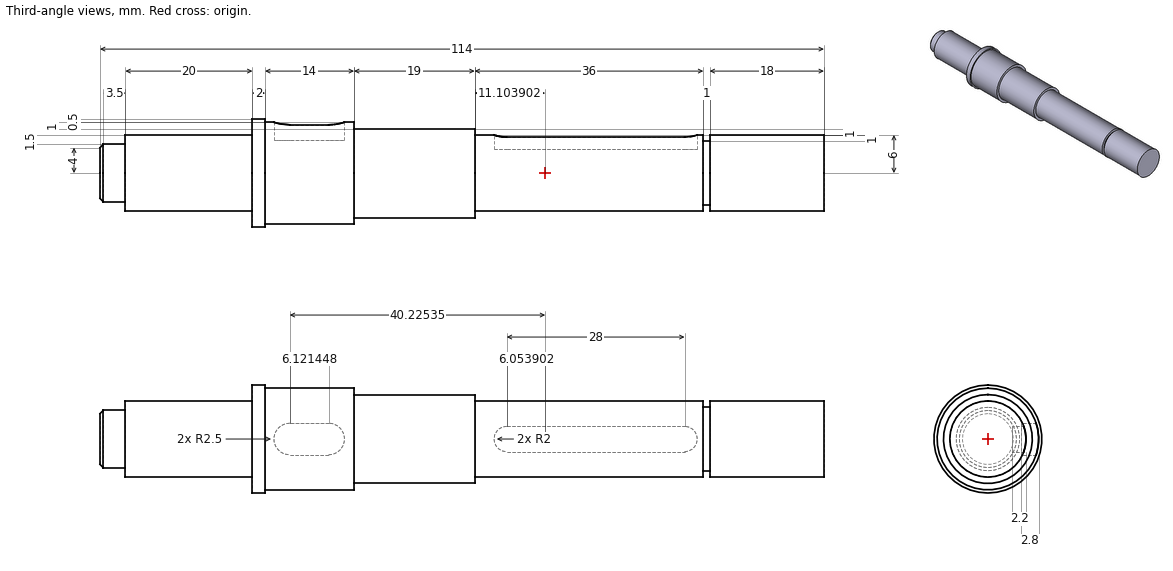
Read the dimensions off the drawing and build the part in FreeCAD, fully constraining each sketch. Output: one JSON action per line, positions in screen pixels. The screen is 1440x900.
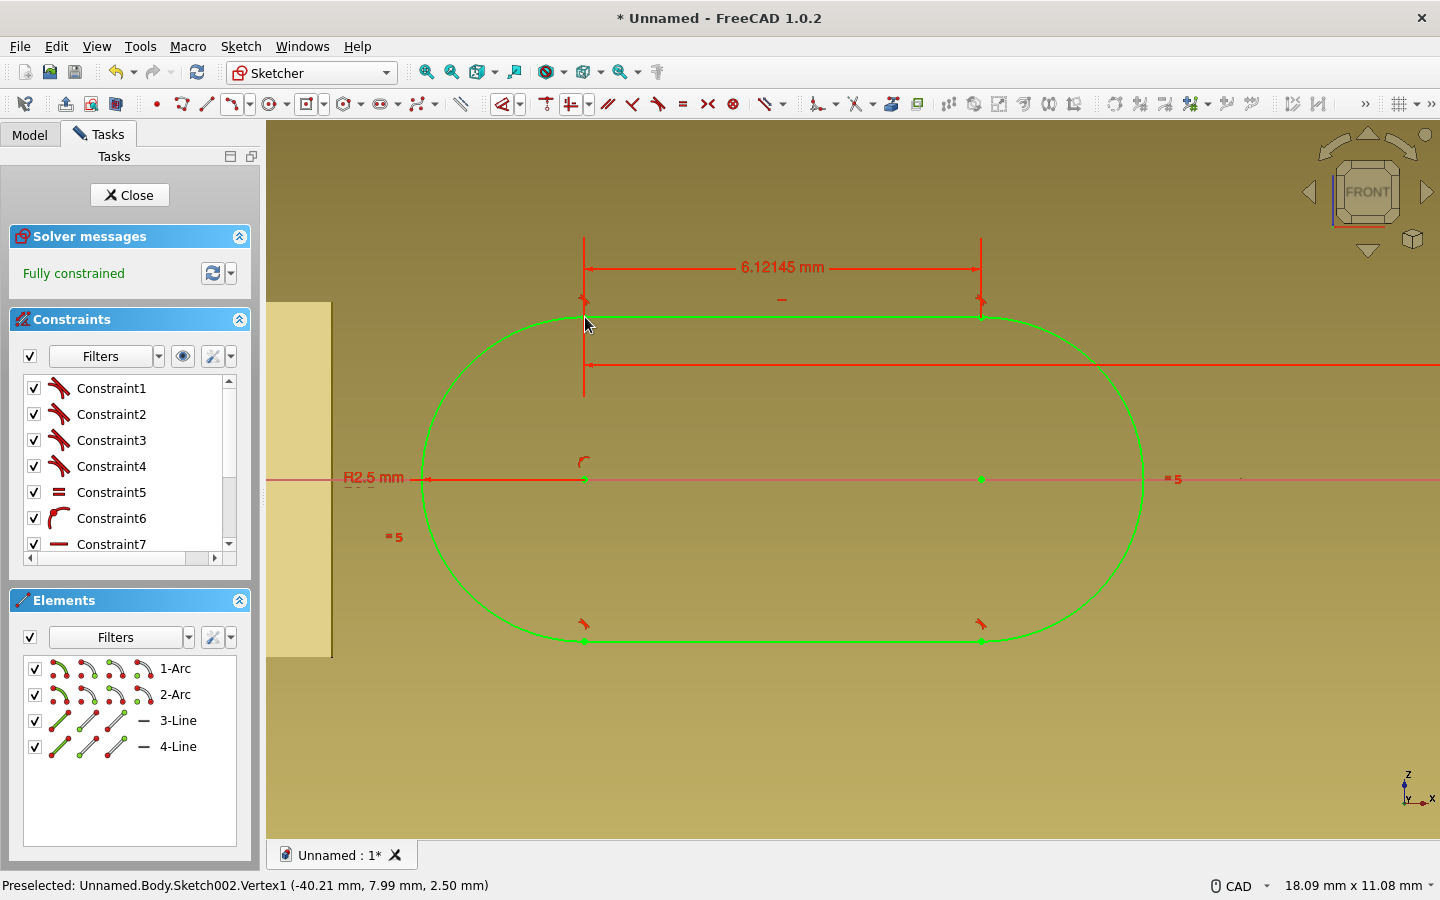
{"action": "left_click", "coordinate": [130, 195]}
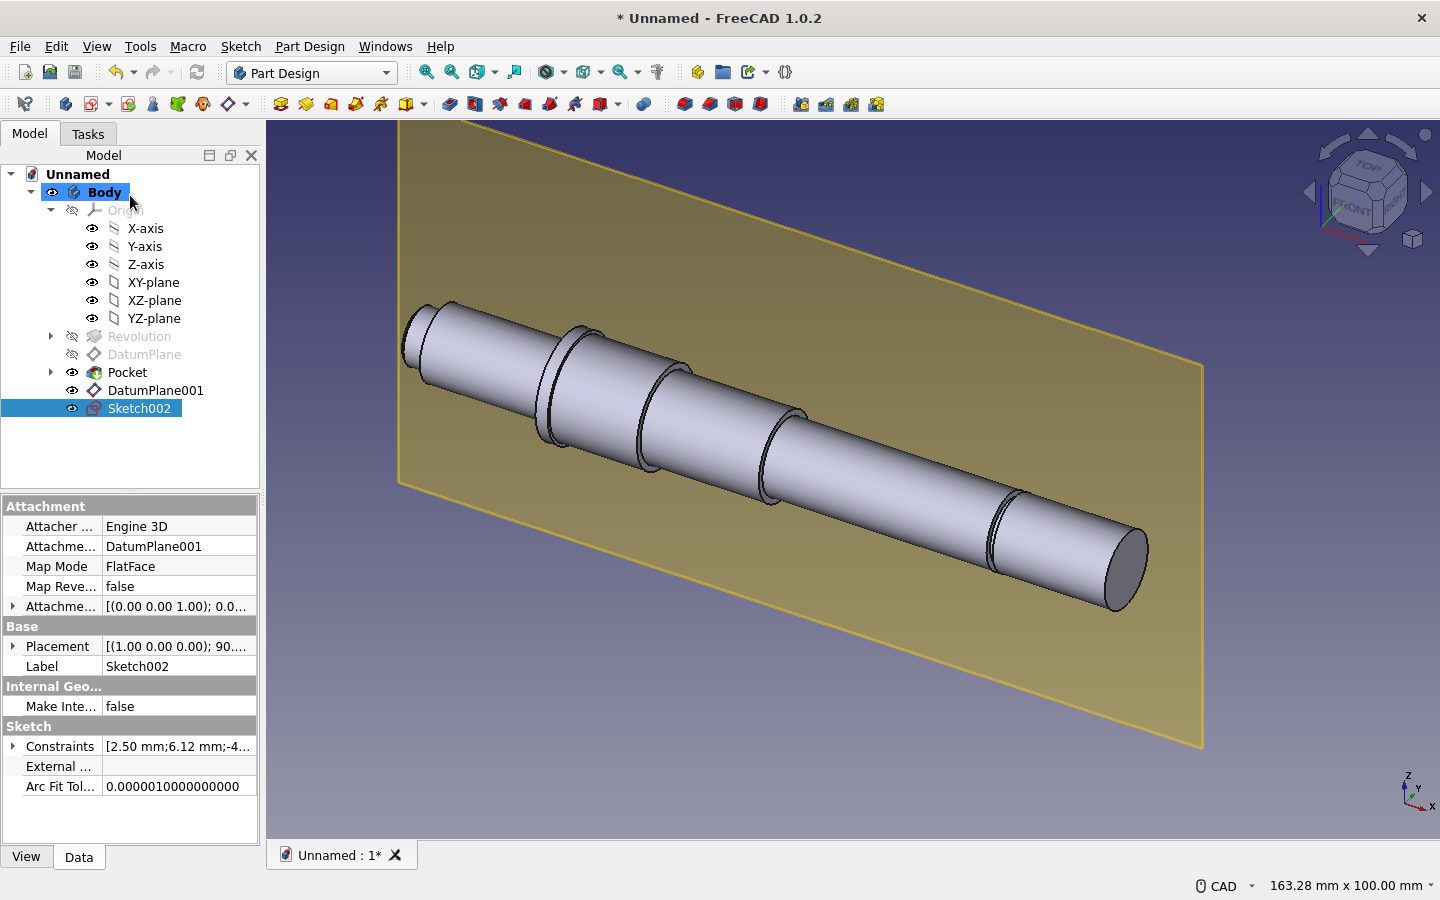
{"action": "left_click", "coordinate": [450, 104]}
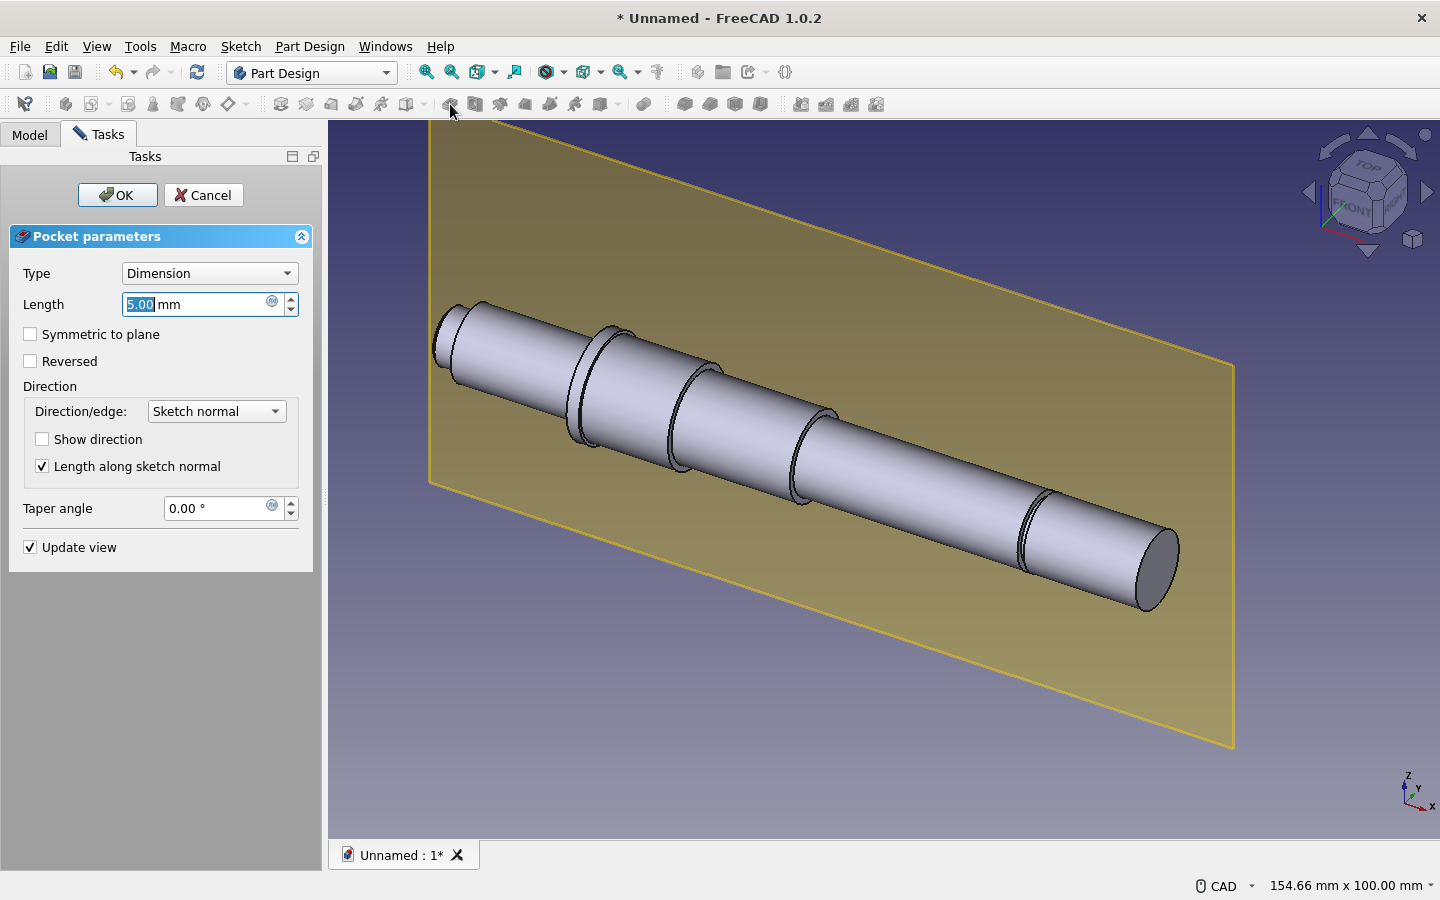
{"action": "type", "text": "2.8"}
{"action": "key", "text": "Tab"}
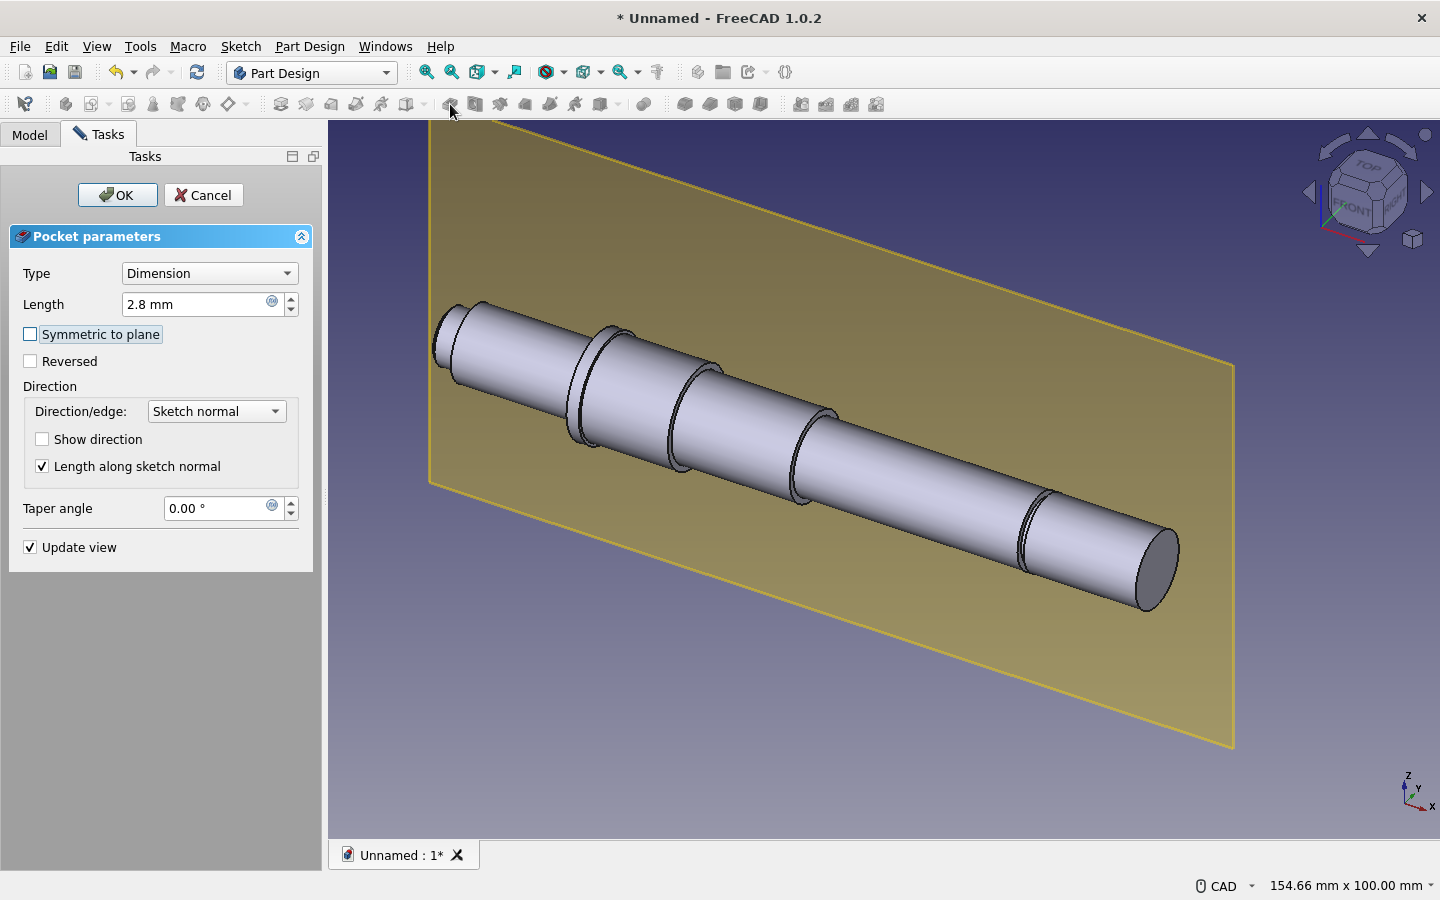
{"action": "left_click", "coordinate": [31, 361]}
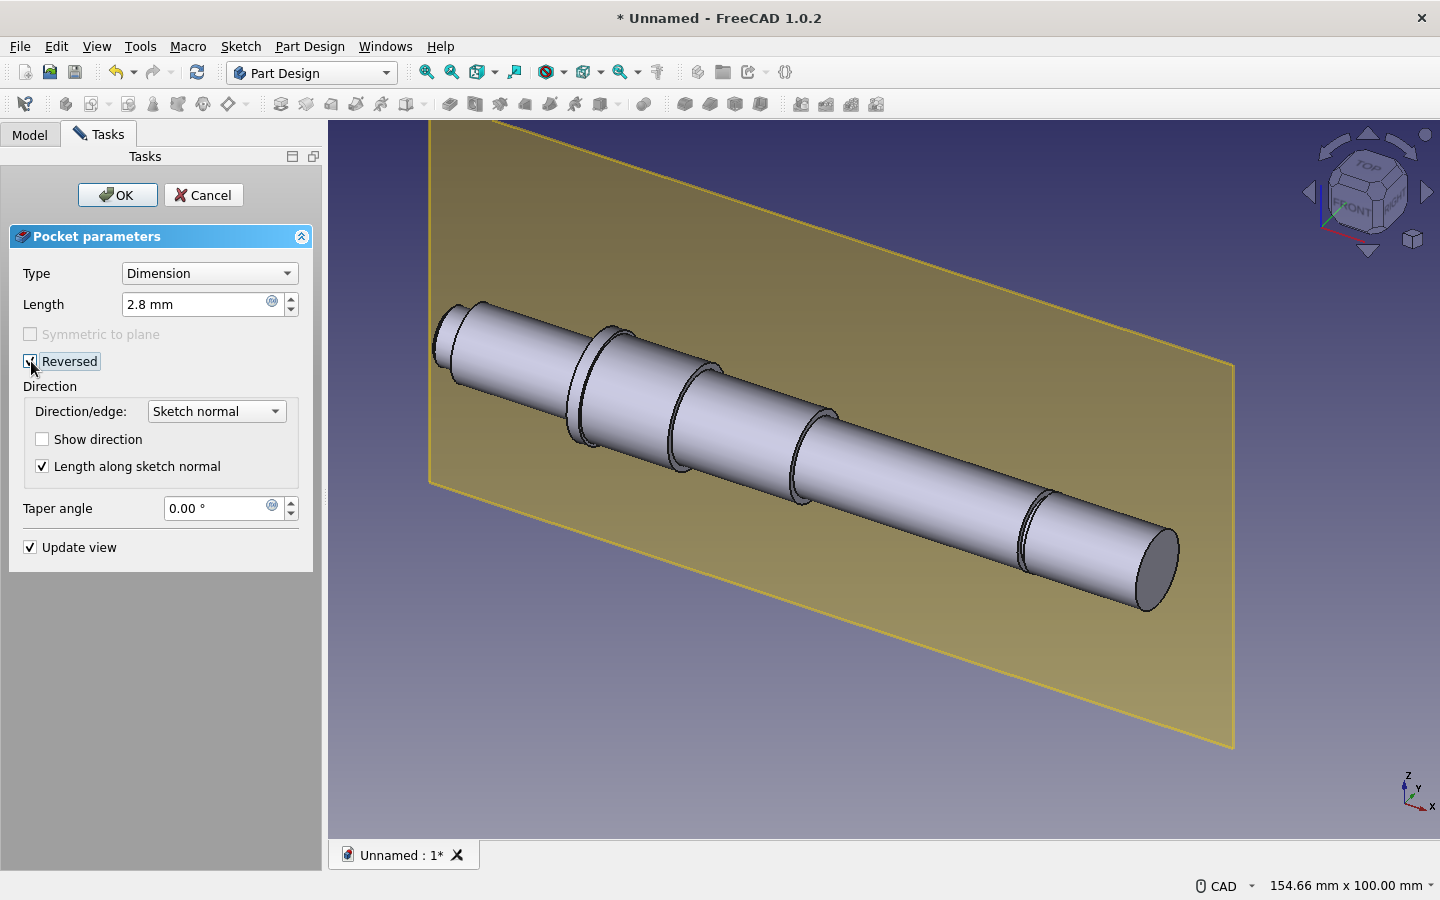
{"action": "left_click", "coordinate": [118, 195]}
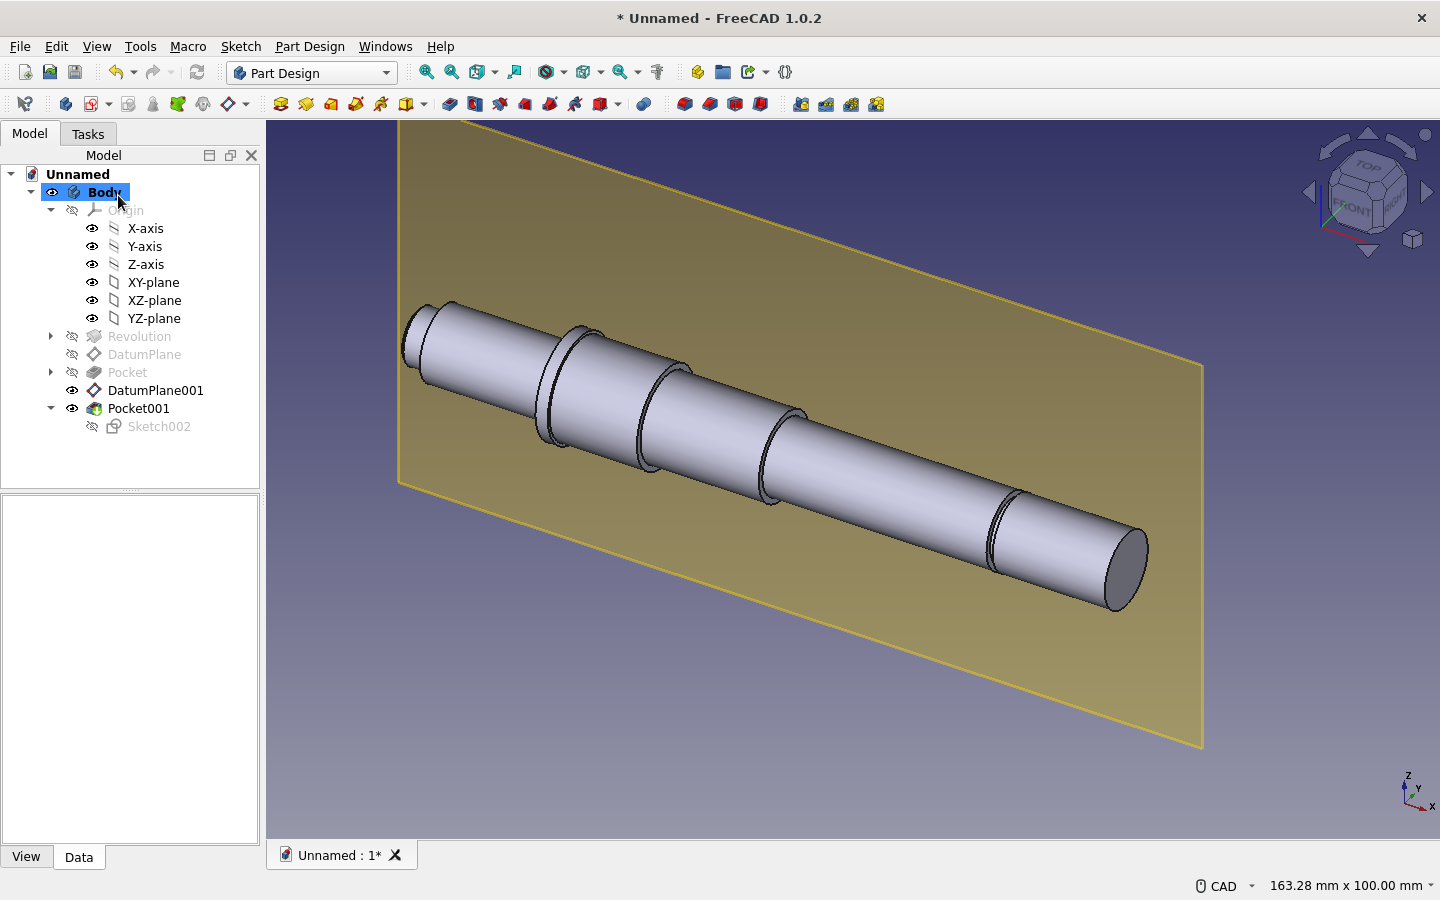
{"action": "left_click", "coordinate": [117, 390]}
{"action": "key", "text": "space"}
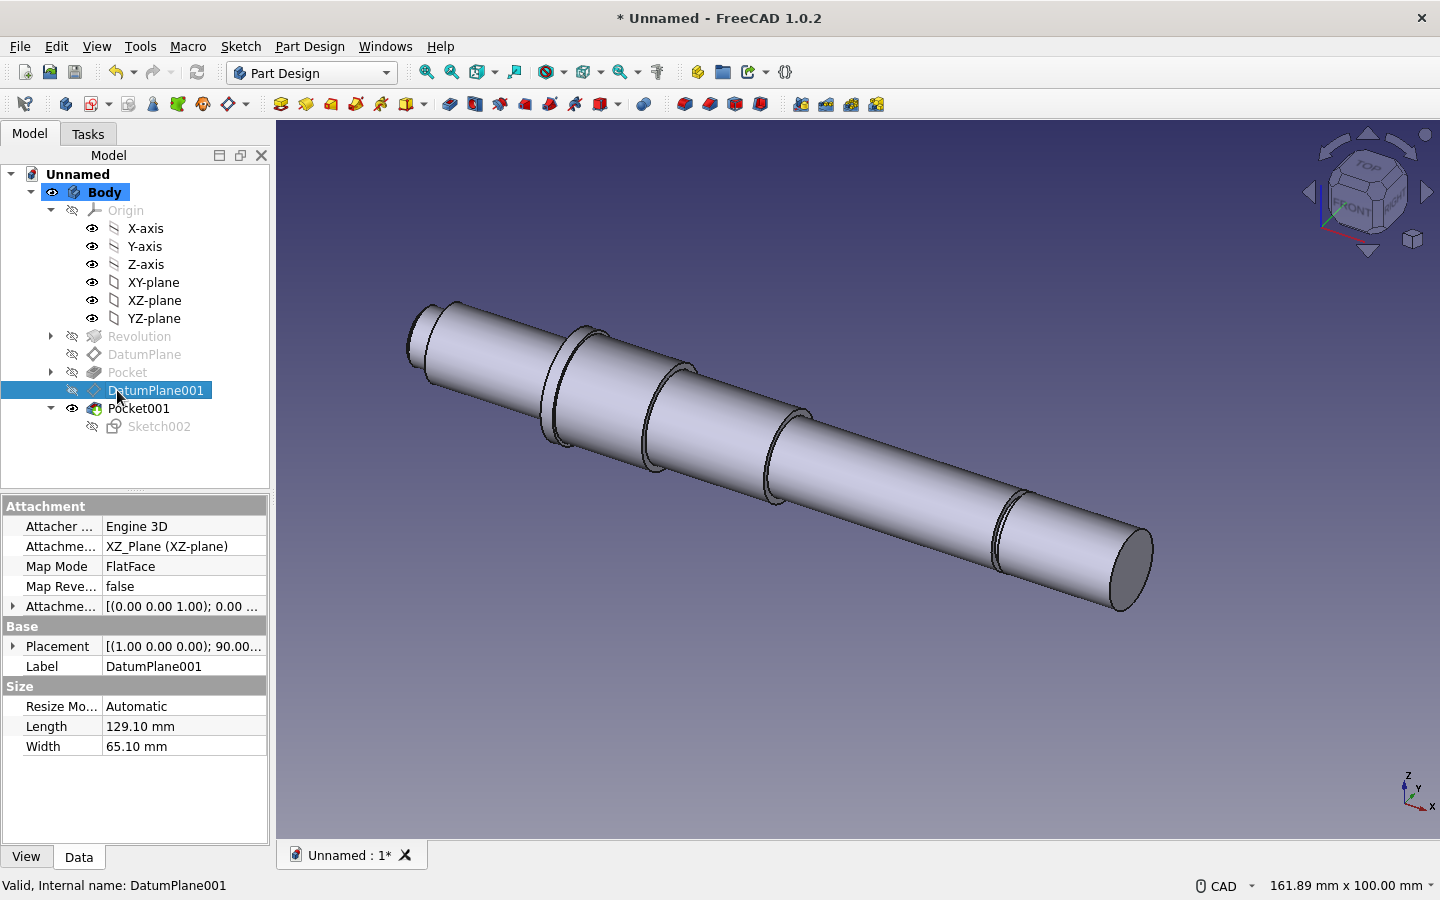
{"action": "key", "text": "0"}